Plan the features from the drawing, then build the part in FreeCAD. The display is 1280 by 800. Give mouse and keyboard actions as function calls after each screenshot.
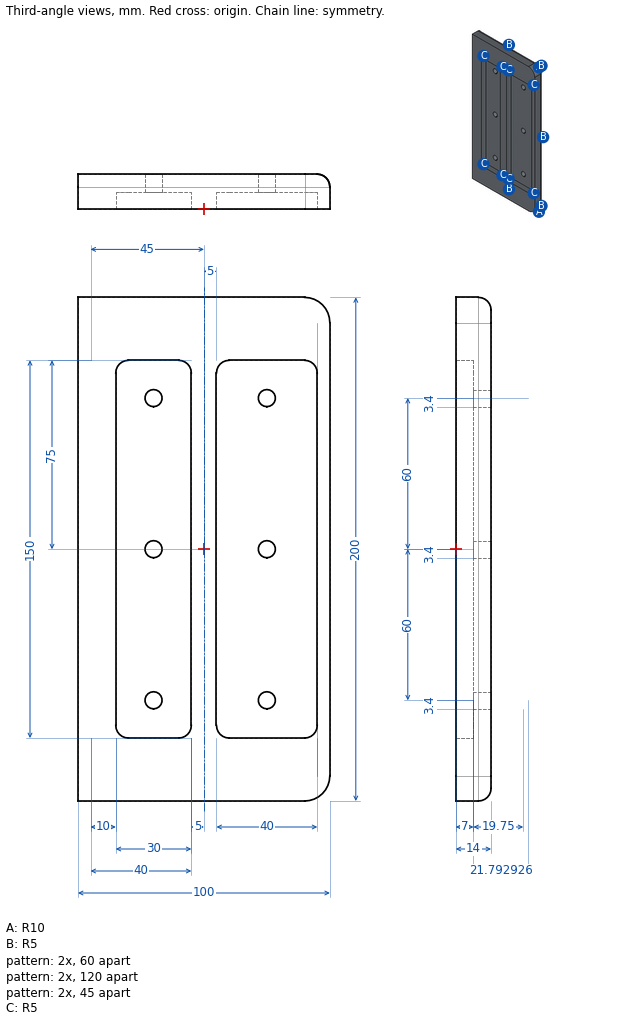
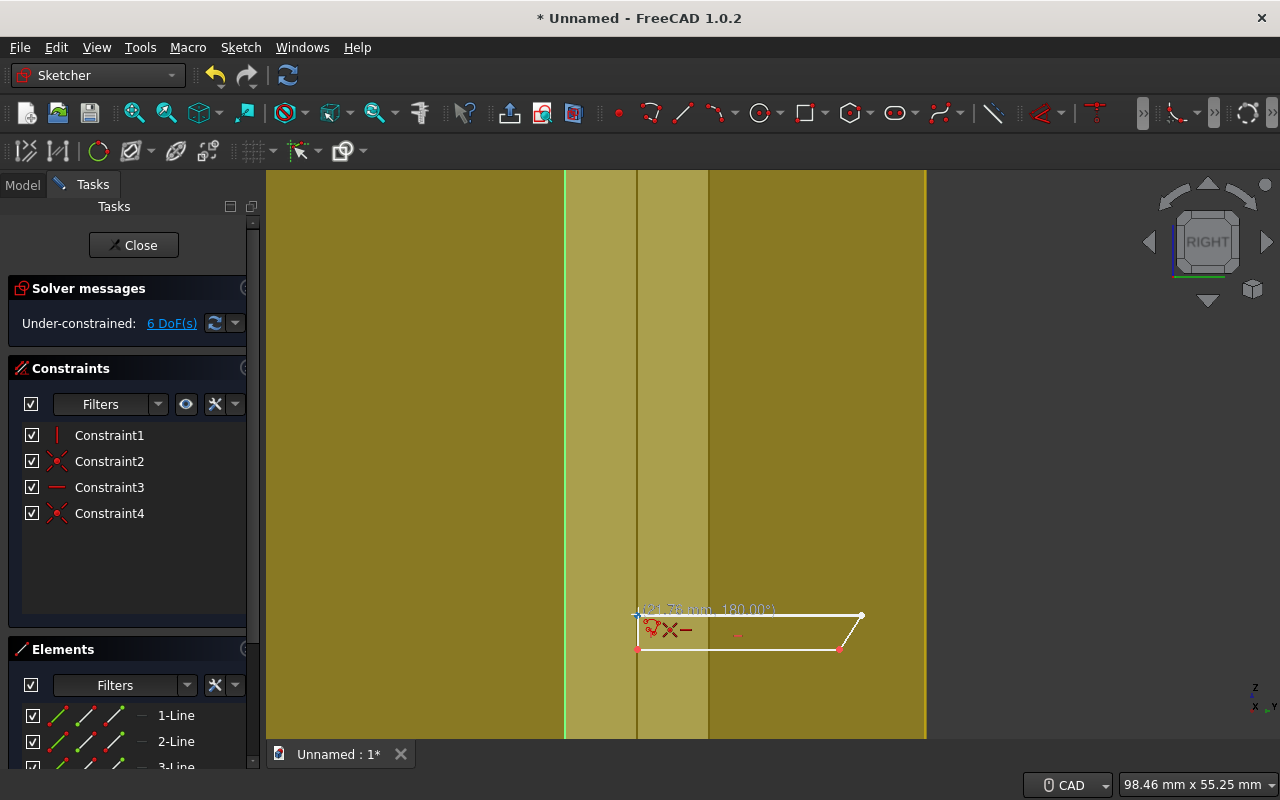
click(638, 615)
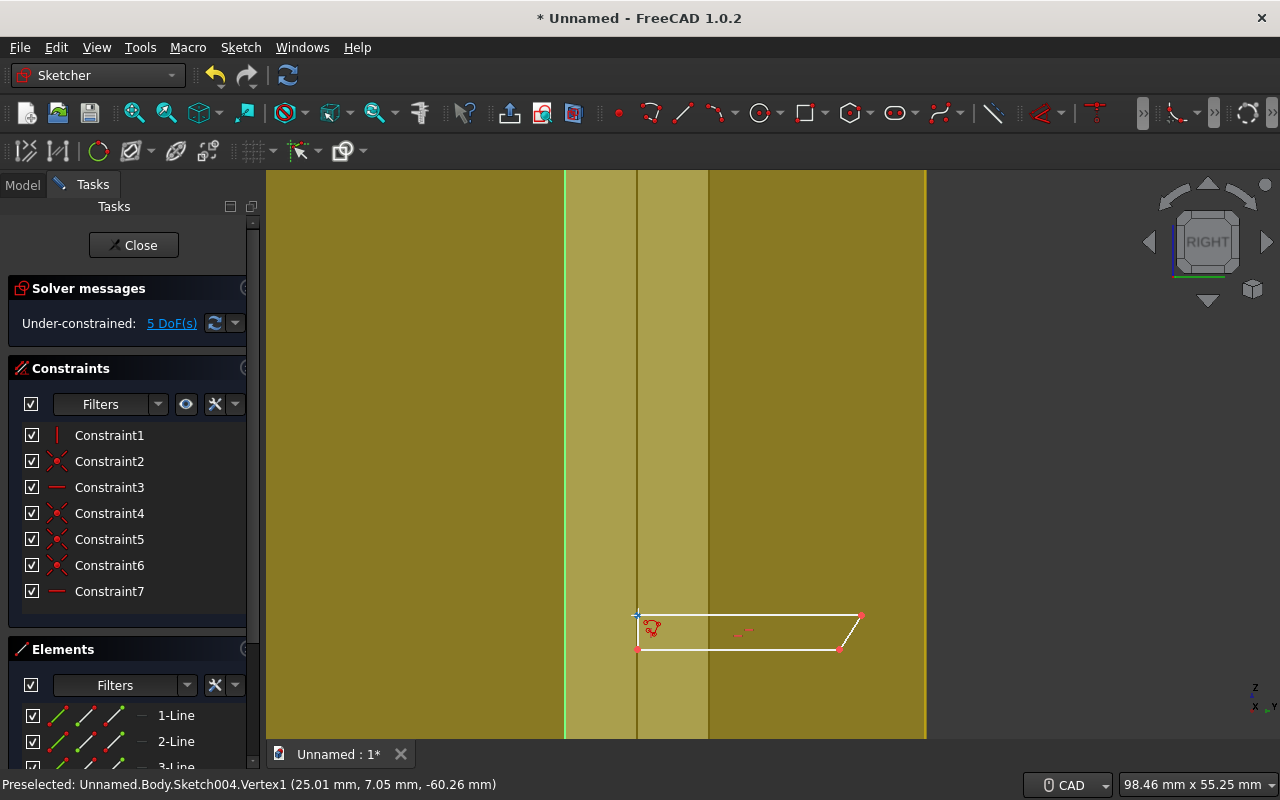
key(g)
key(l)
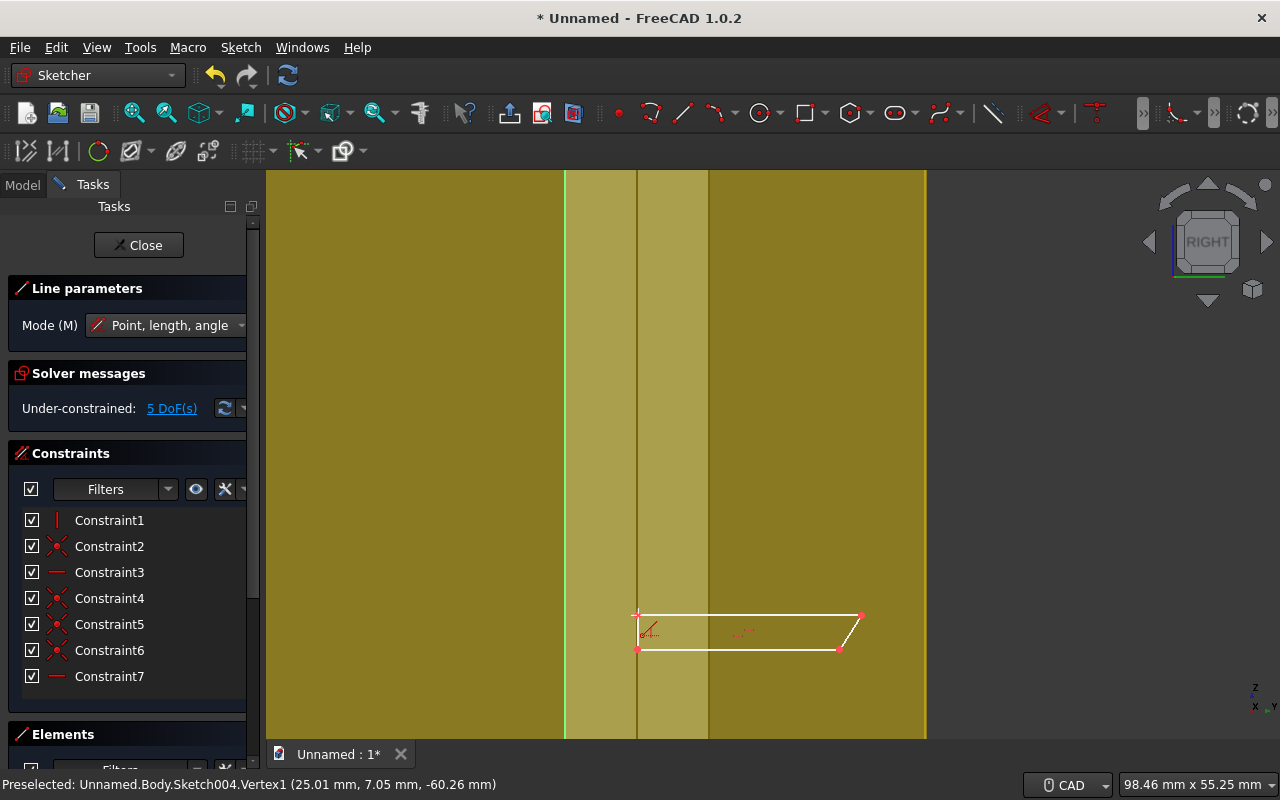
click(884, 613)
click(951, 613)
key(Escape)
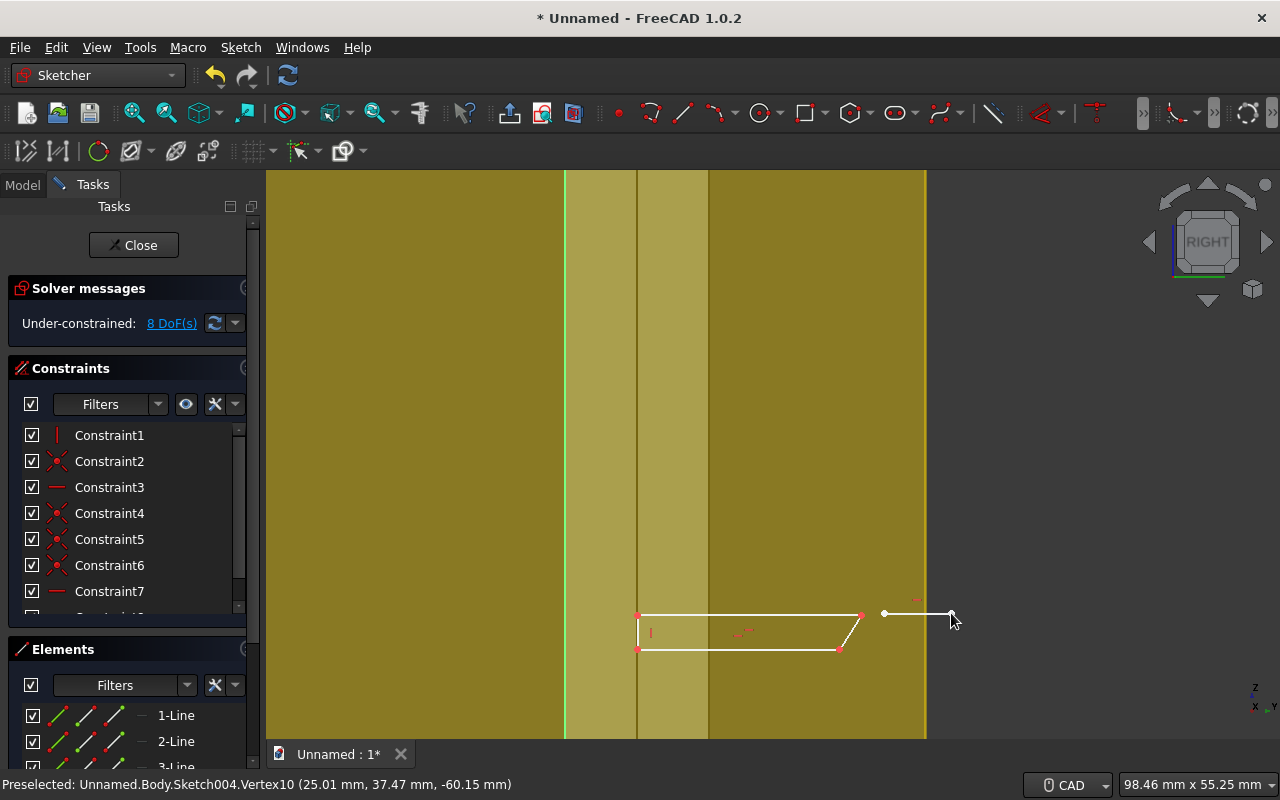
click(904, 614)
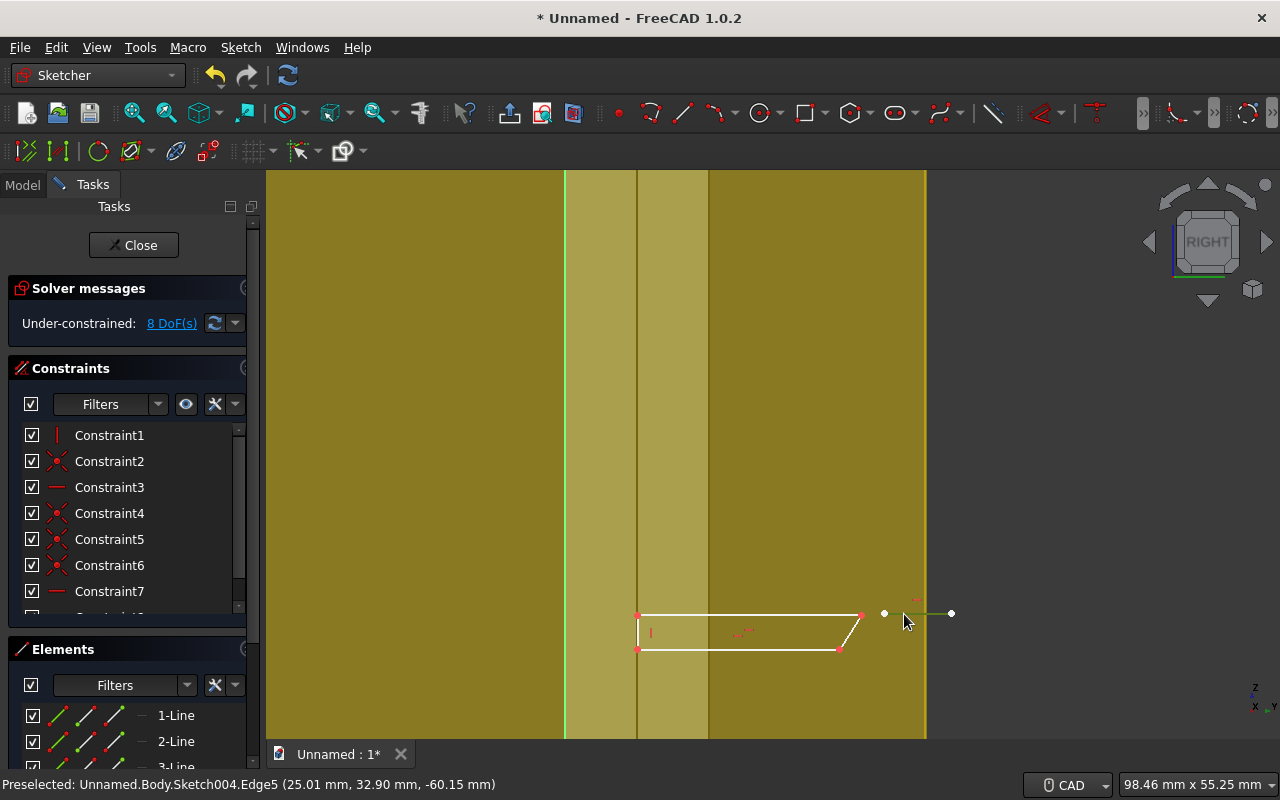
click(994, 114)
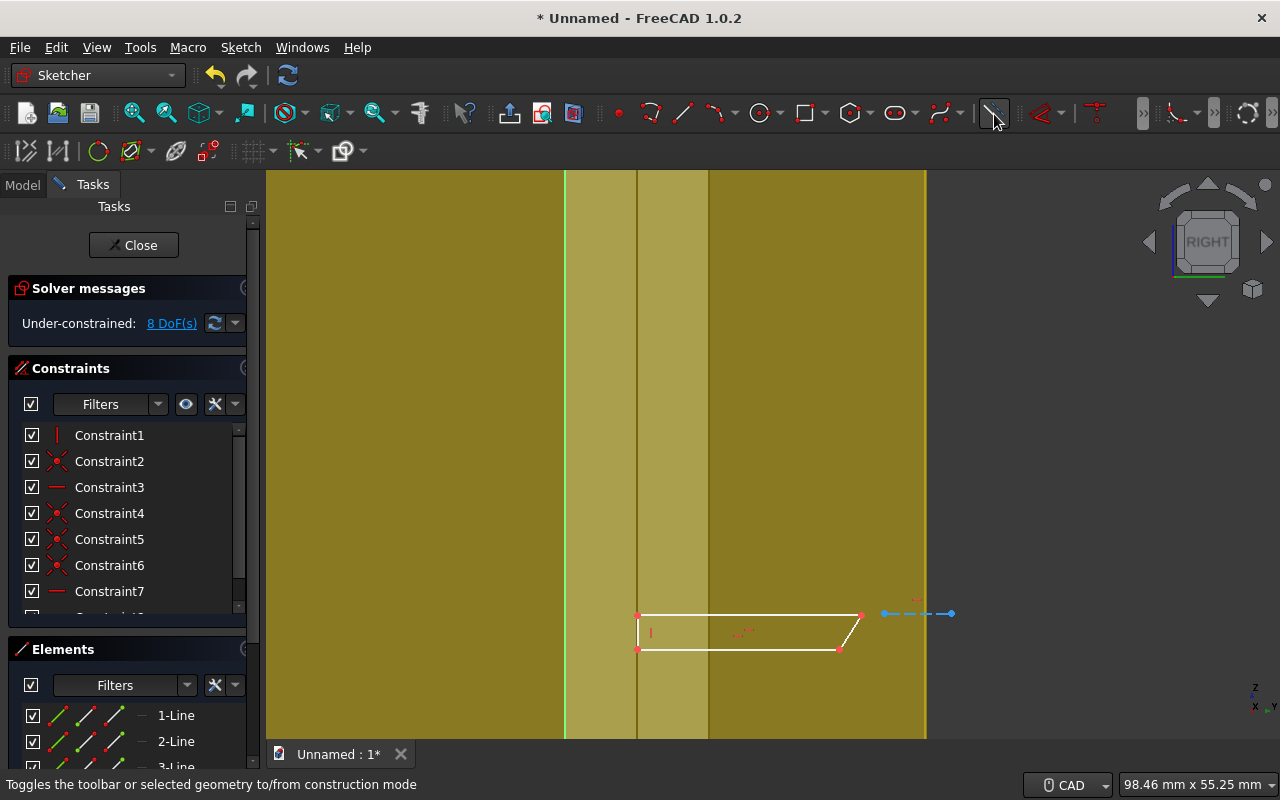
click(1040, 114)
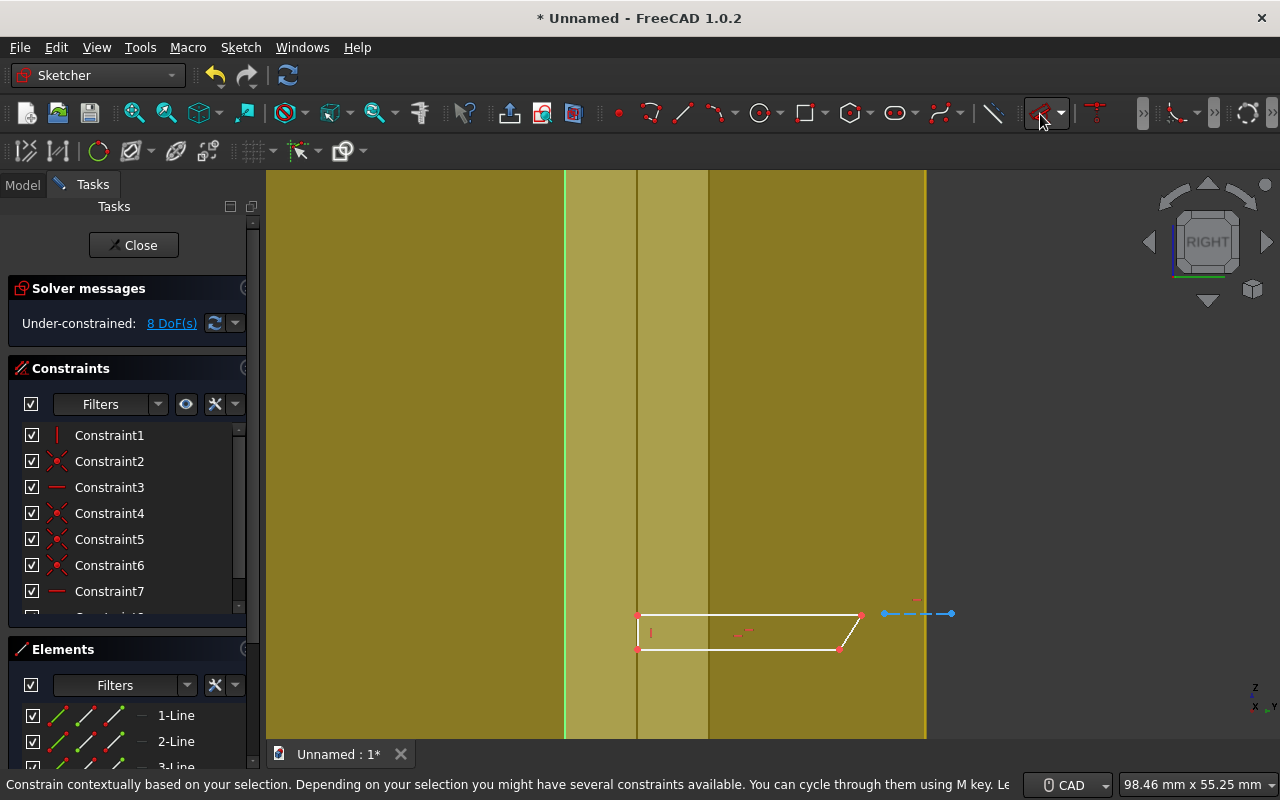
click(638, 615)
click(601, 649)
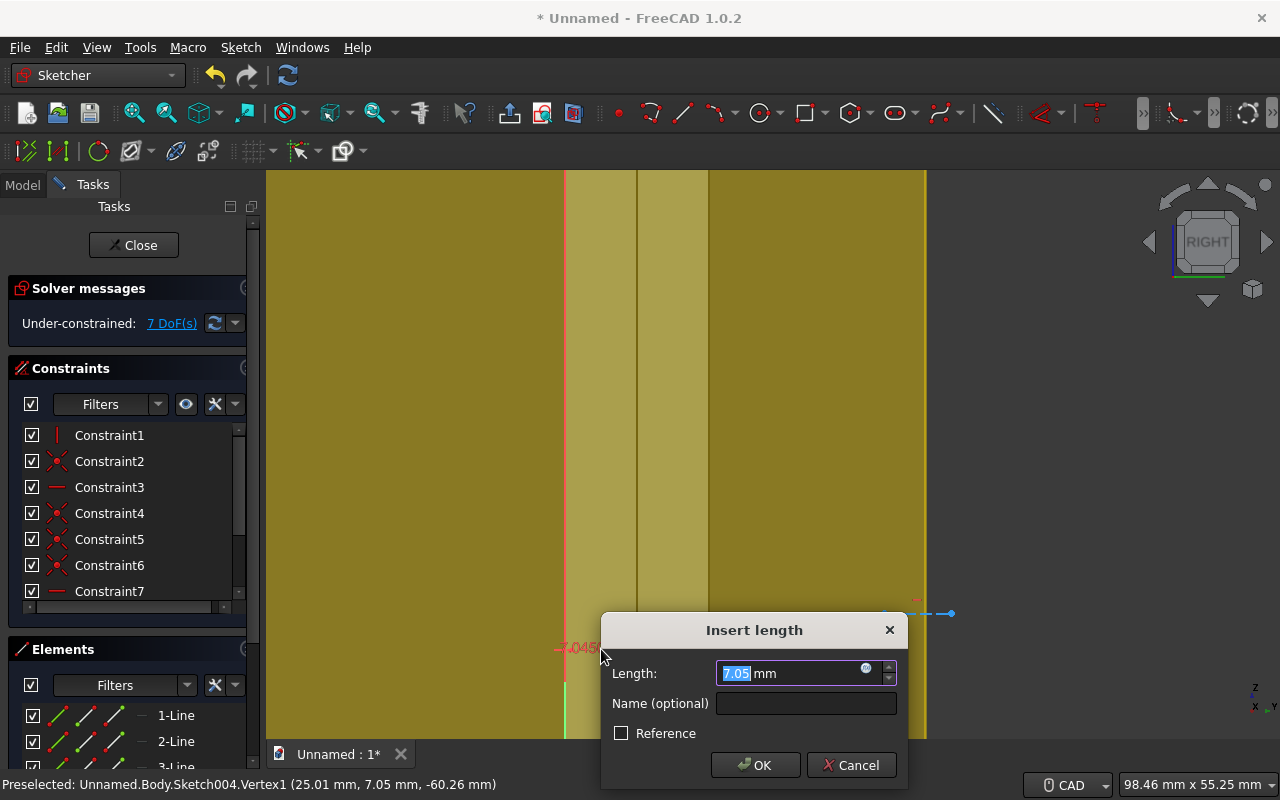
text(7)
key(Return)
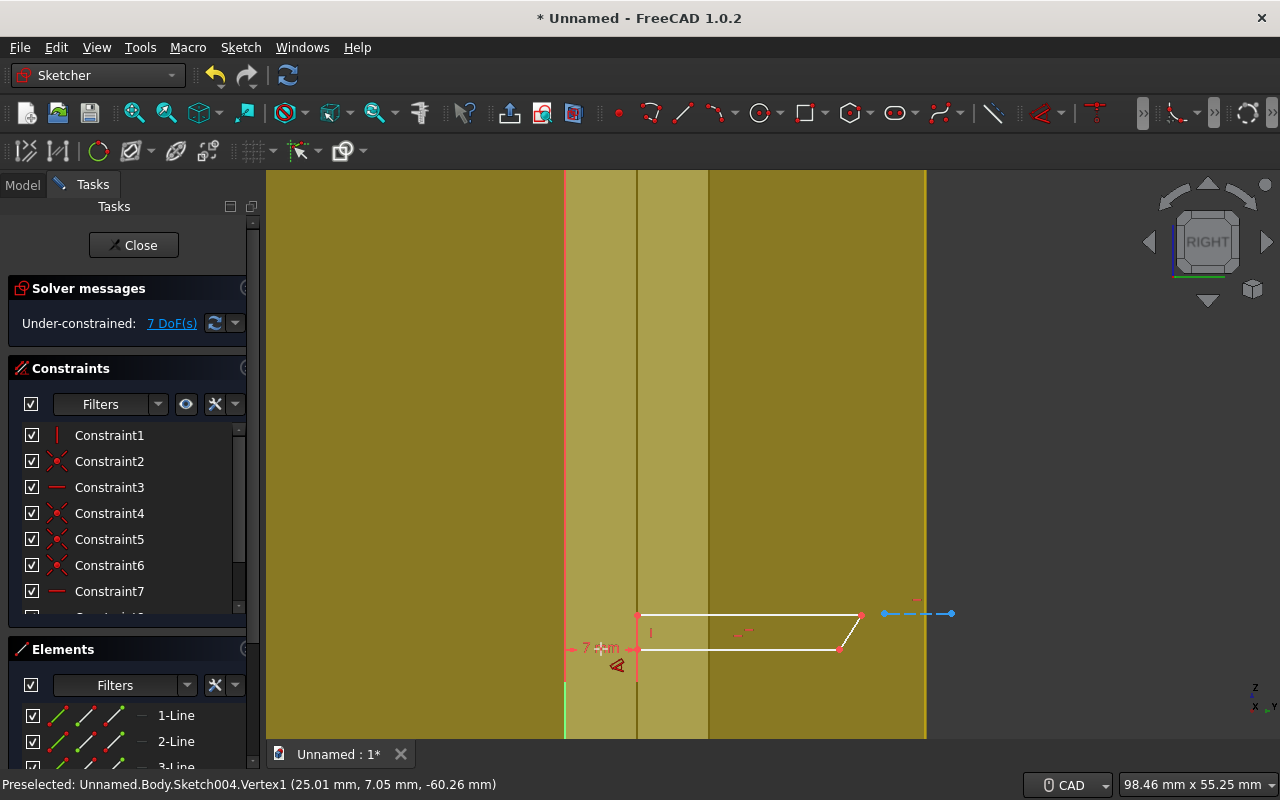
scroll(637, 626, up, 2)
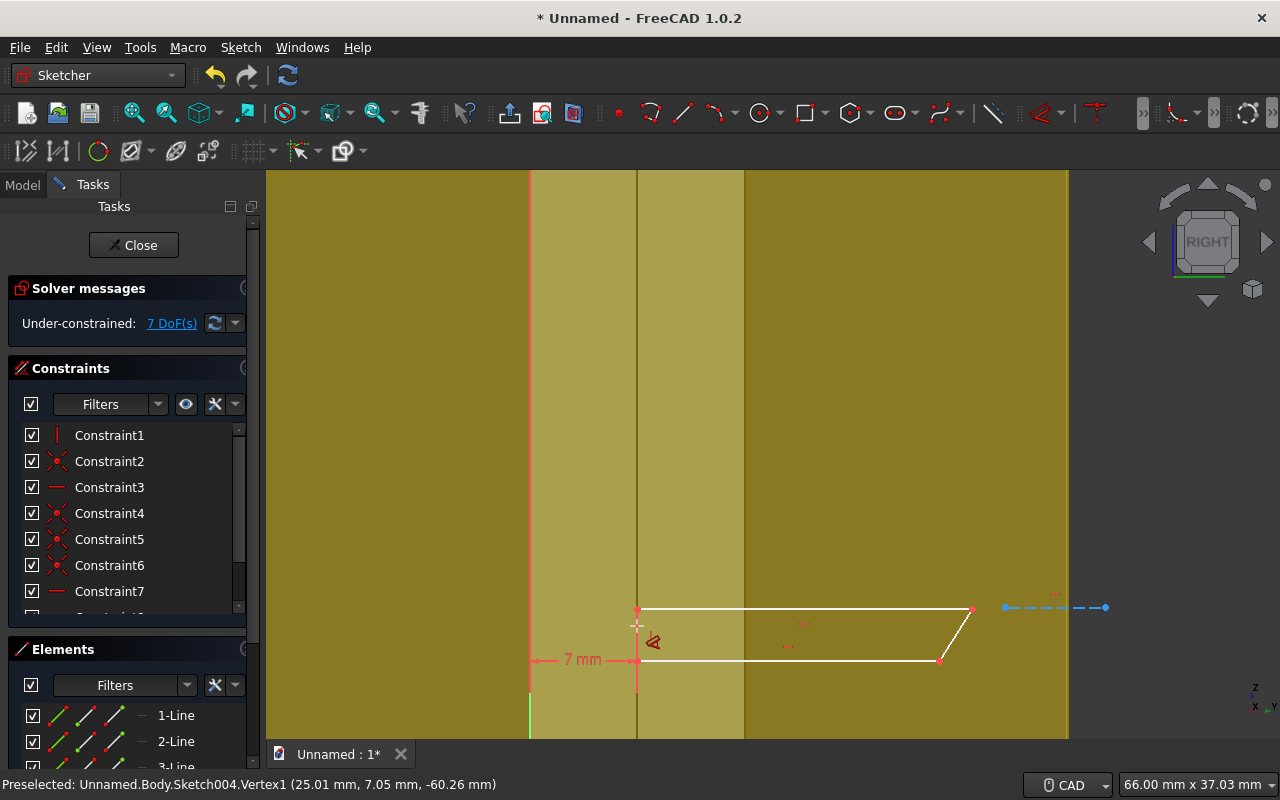
click(637, 625)
click(603, 635)